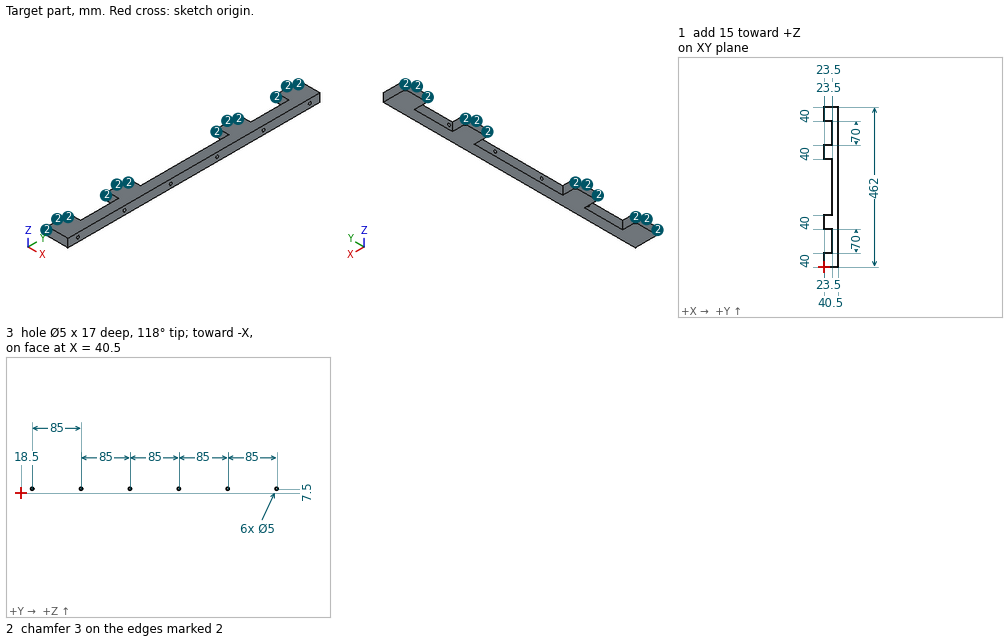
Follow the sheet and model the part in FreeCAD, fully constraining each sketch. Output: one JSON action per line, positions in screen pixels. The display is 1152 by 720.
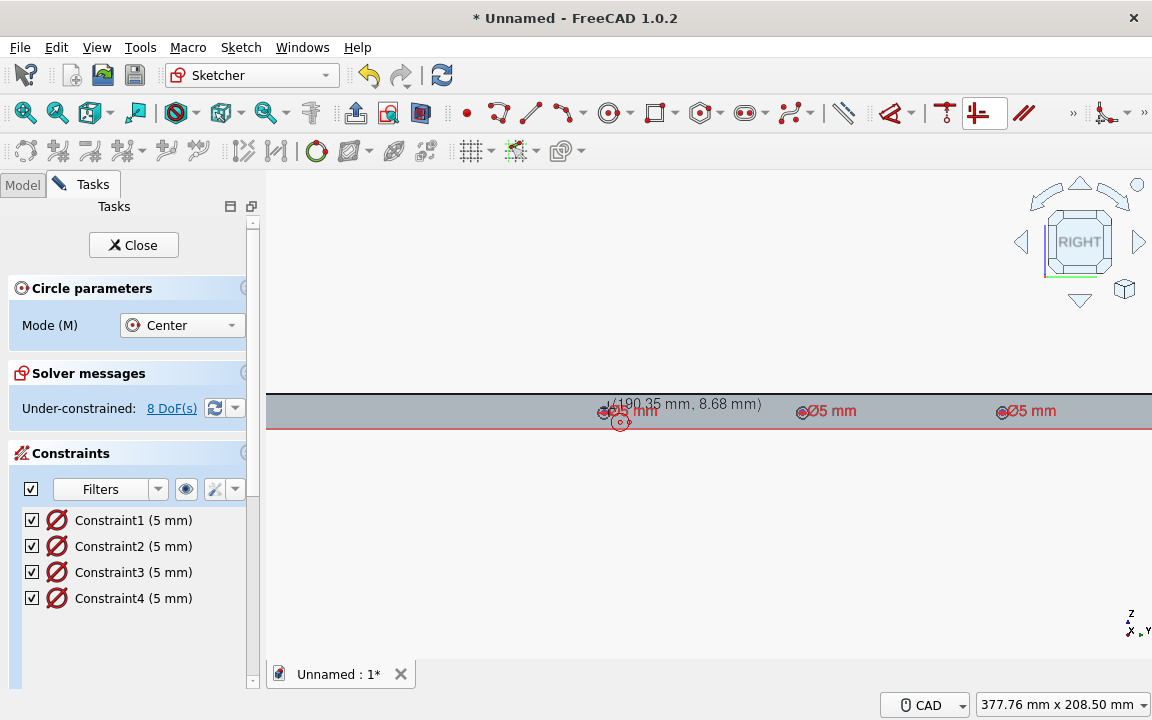
{"action": "scroll", "coordinate": [404, 412], "scroll_direction": "up", "scroll_amount": 7}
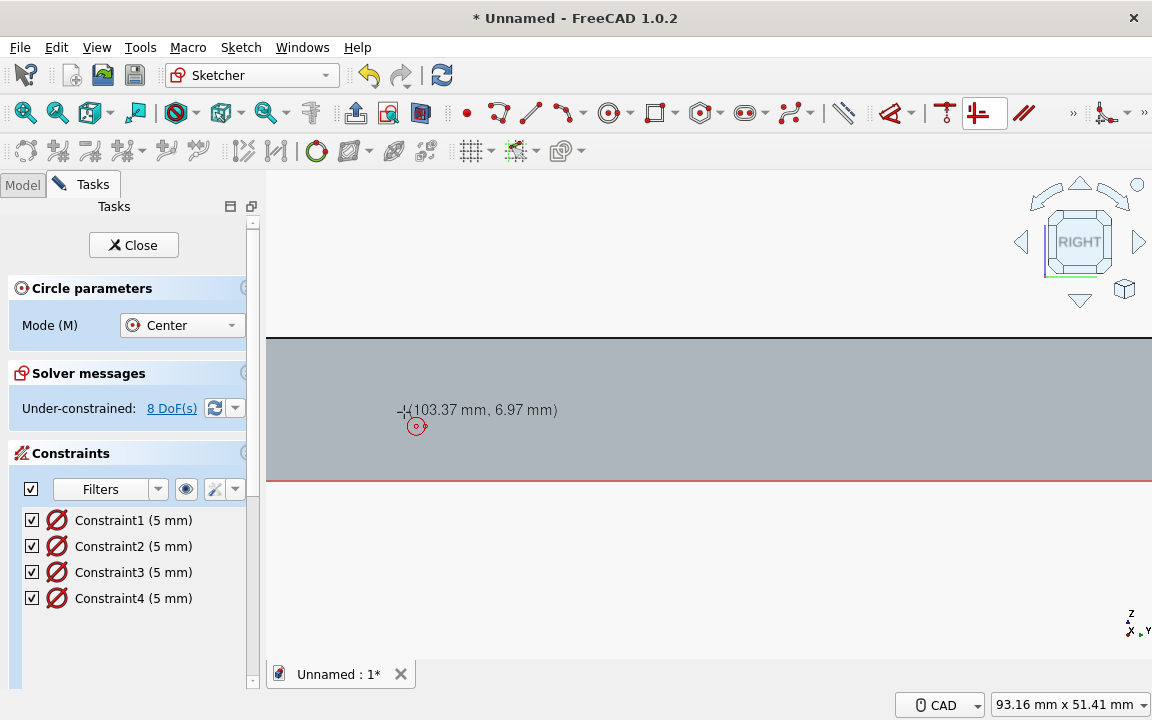
{"action": "scroll", "coordinate": [528, 412], "scroll_direction": "down", "scroll_amount": 11}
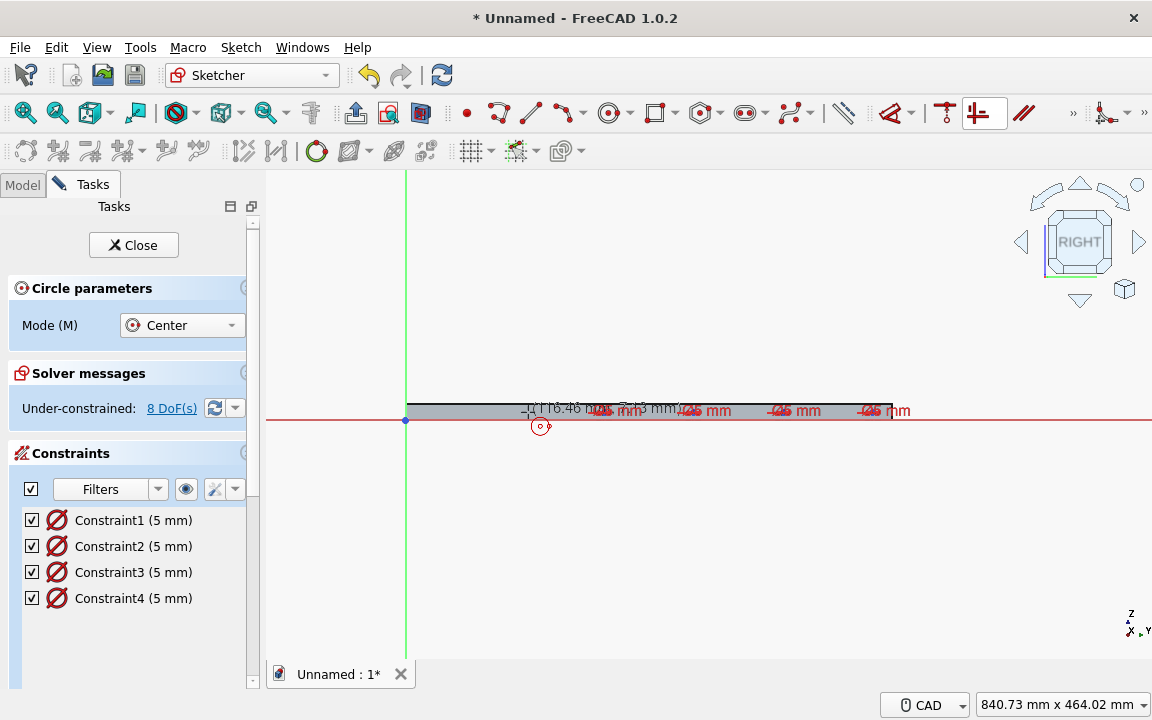
{"action": "scroll", "coordinate": [515, 412], "scroll_direction": "up", "scroll_amount": 4}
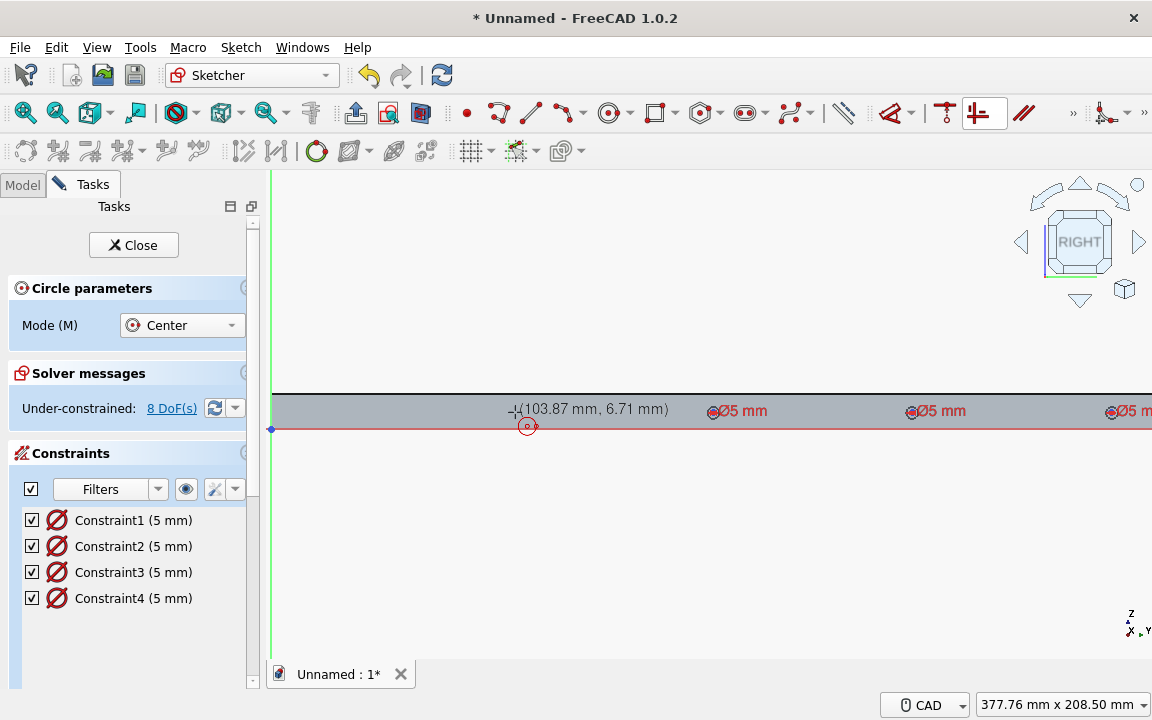
{"action": "left_click", "coordinate": [514, 412]}
{"action": "mouse_move", "coordinate": [518, 408]}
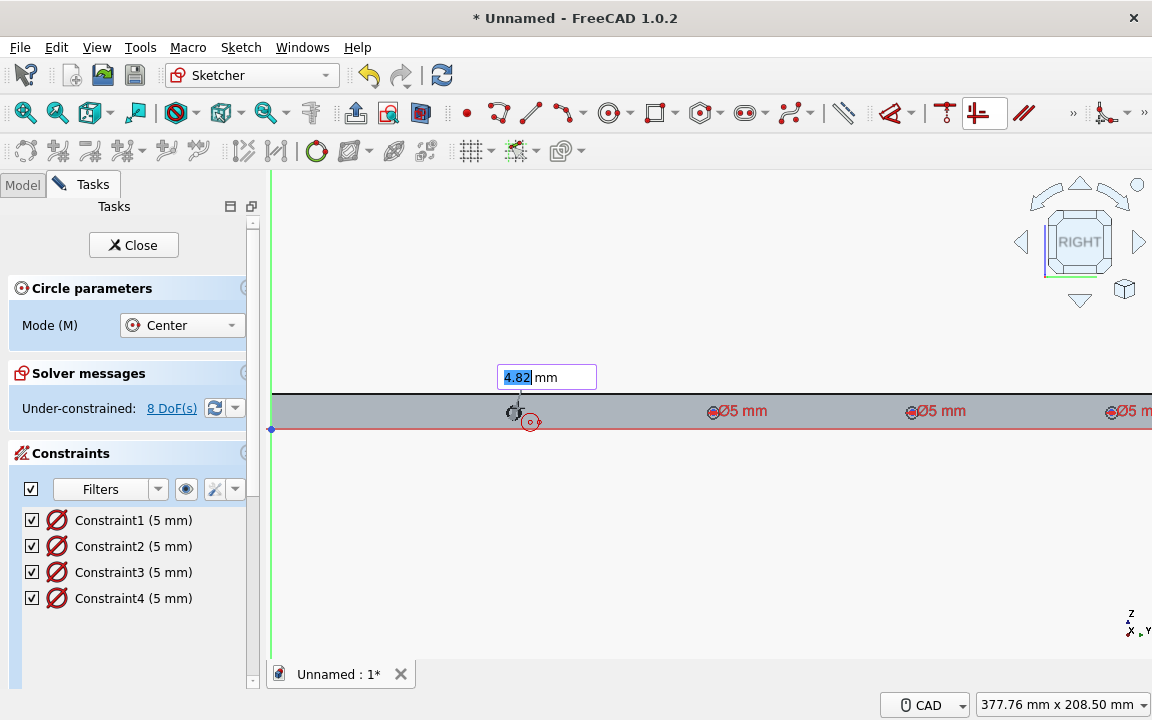
{"action": "type", "text": "5"}
{"action": "key", "text": "Return"}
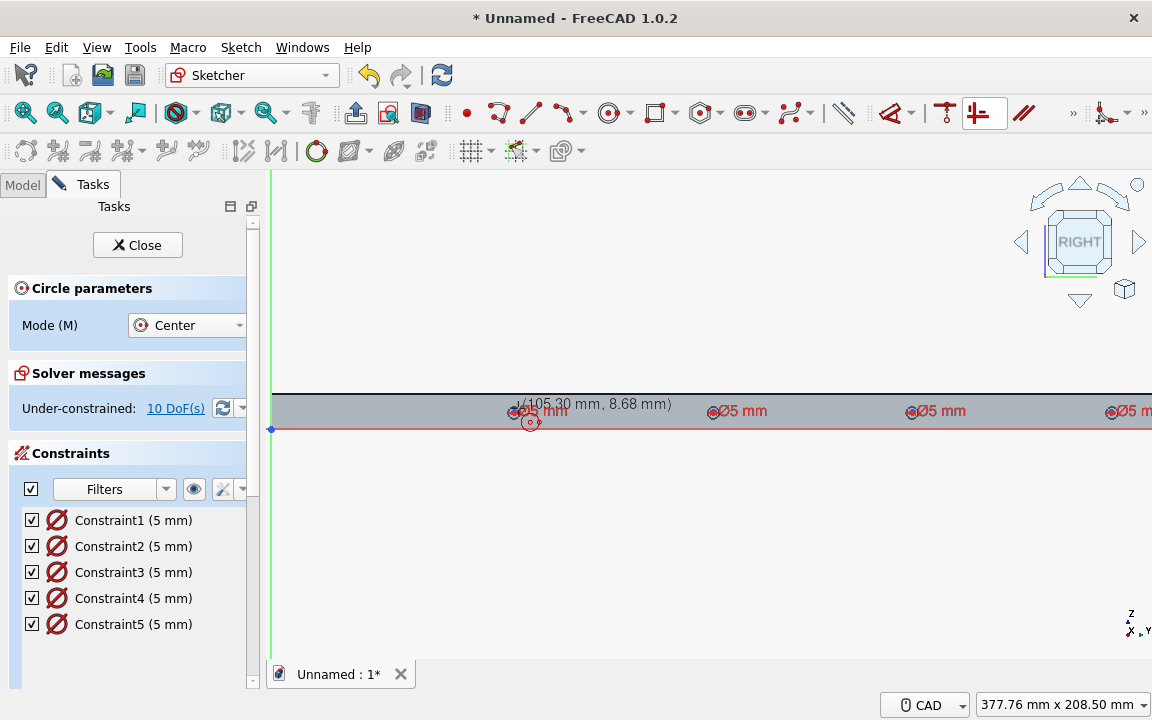
{"action": "scroll", "coordinate": [314, 412], "scroll_direction": "up", "scroll_amount": 7}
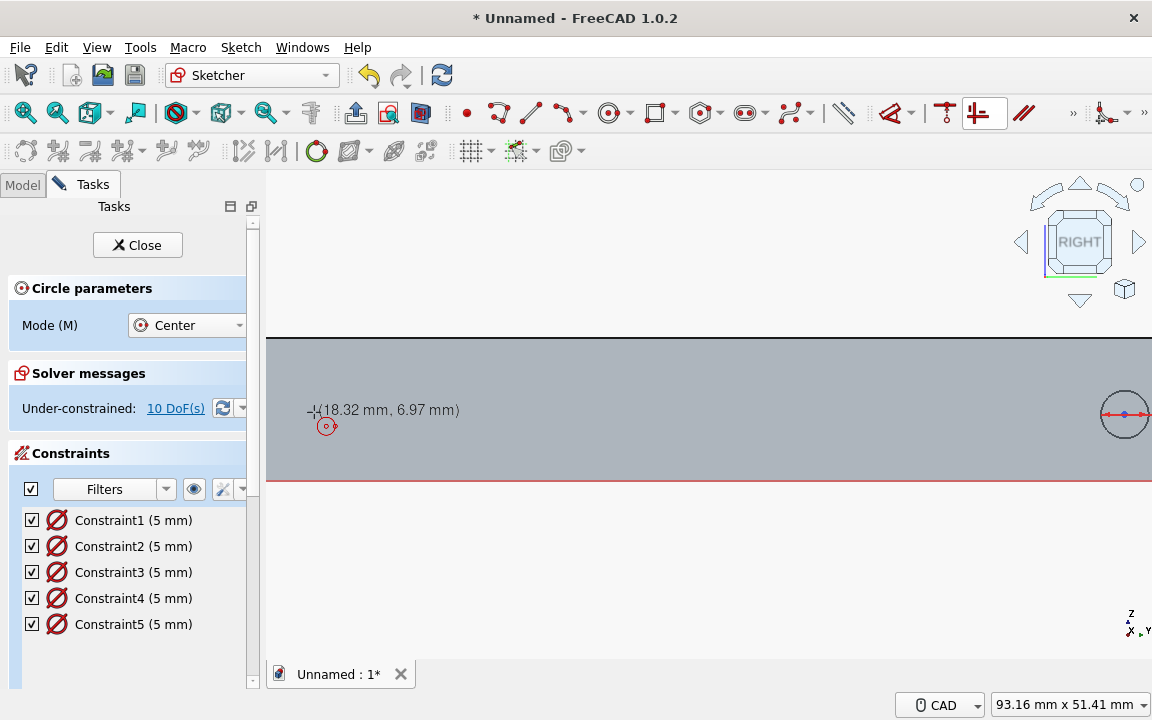
{"action": "scroll", "coordinate": [439, 412], "scroll_direction": "down", "scroll_amount": 11}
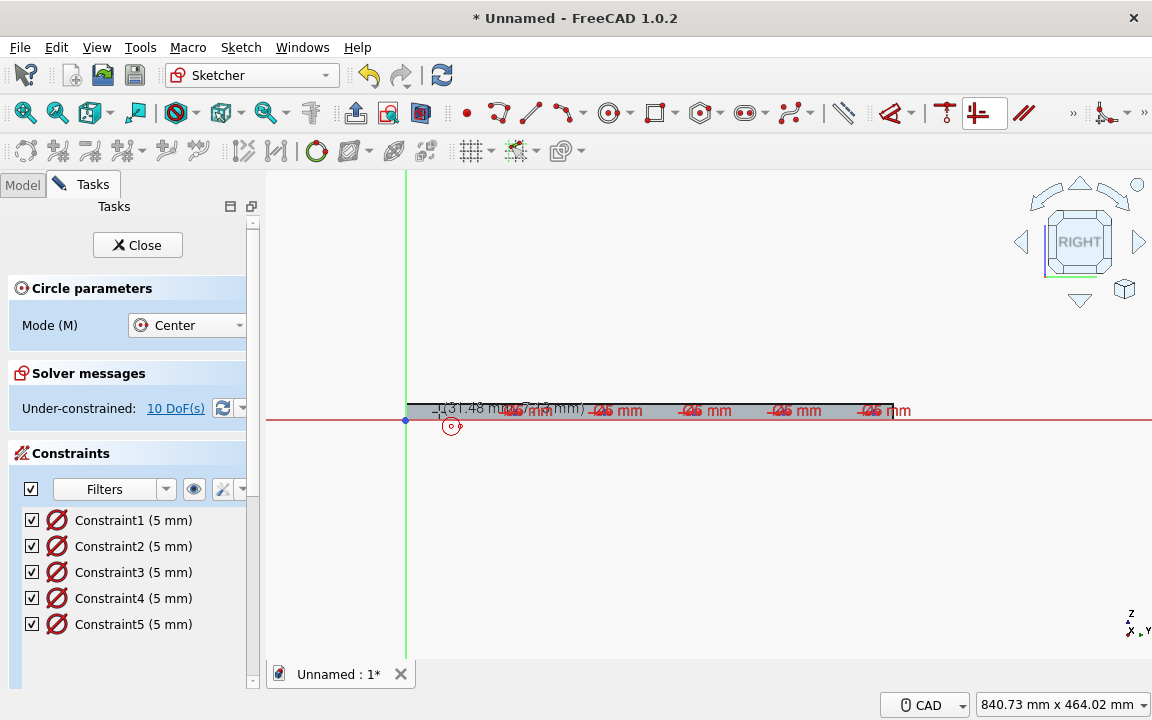
{"action": "scroll", "coordinate": [425, 412], "scroll_direction": "up", "scroll_amount": 4}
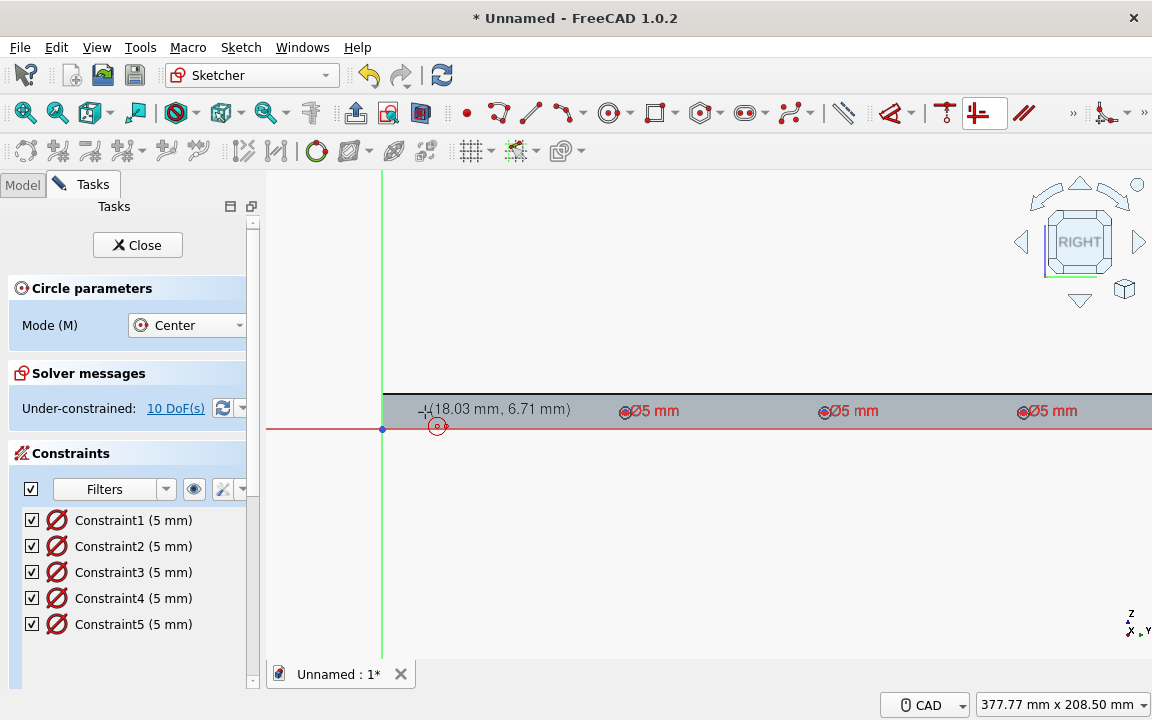
{"action": "left_click", "coordinate": [426, 412]}
{"action": "mouse_move", "coordinate": [430, 408]}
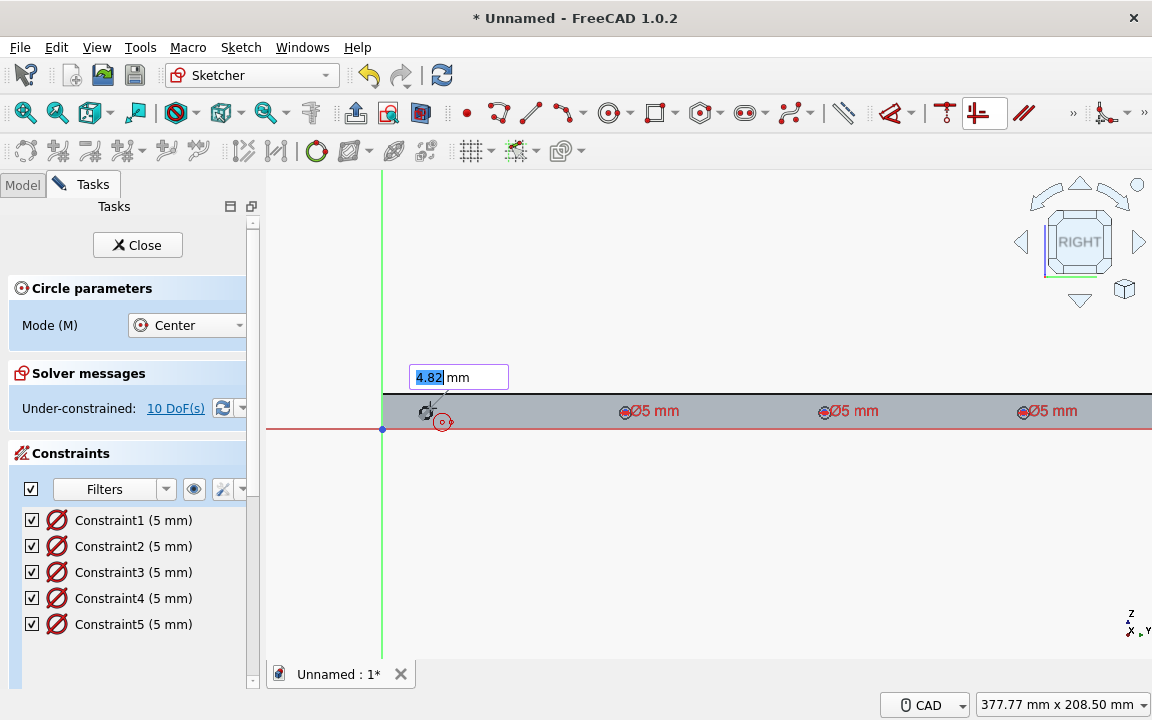
{"action": "type", "text": "5"}
{"action": "key", "text": "Return"}
{"action": "key", "text": "Escape"}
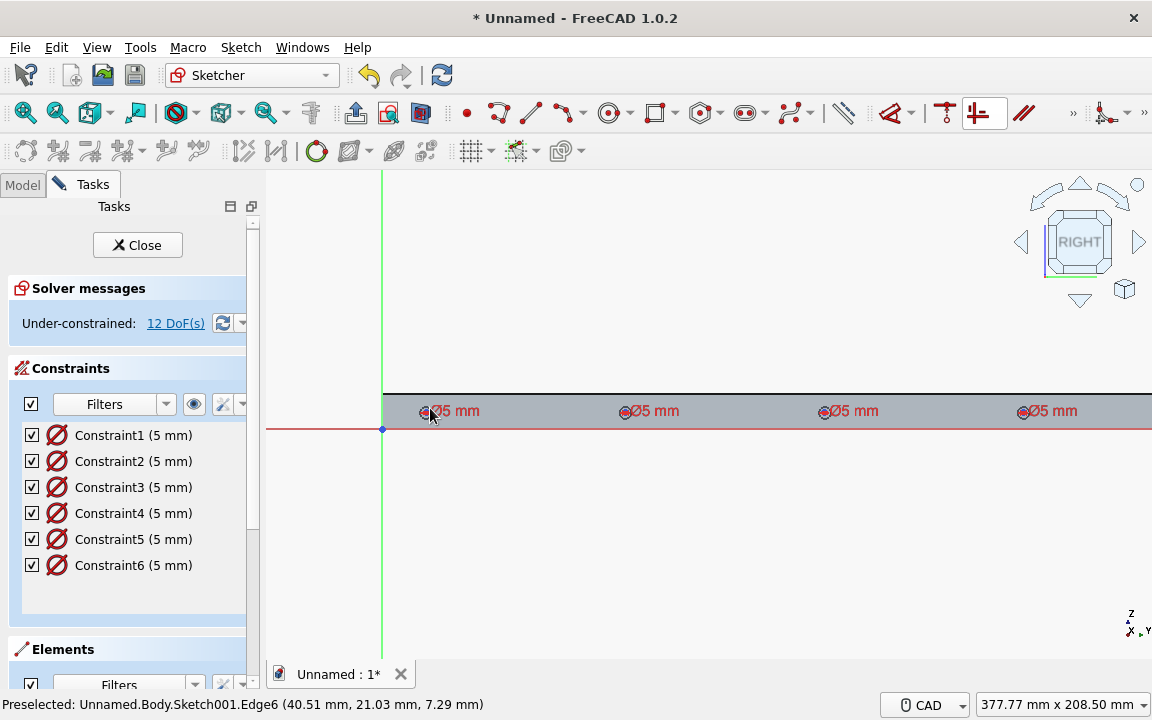
{"action": "scroll", "coordinate": [424, 412], "scroll_direction": "down", "scroll_amount": 4}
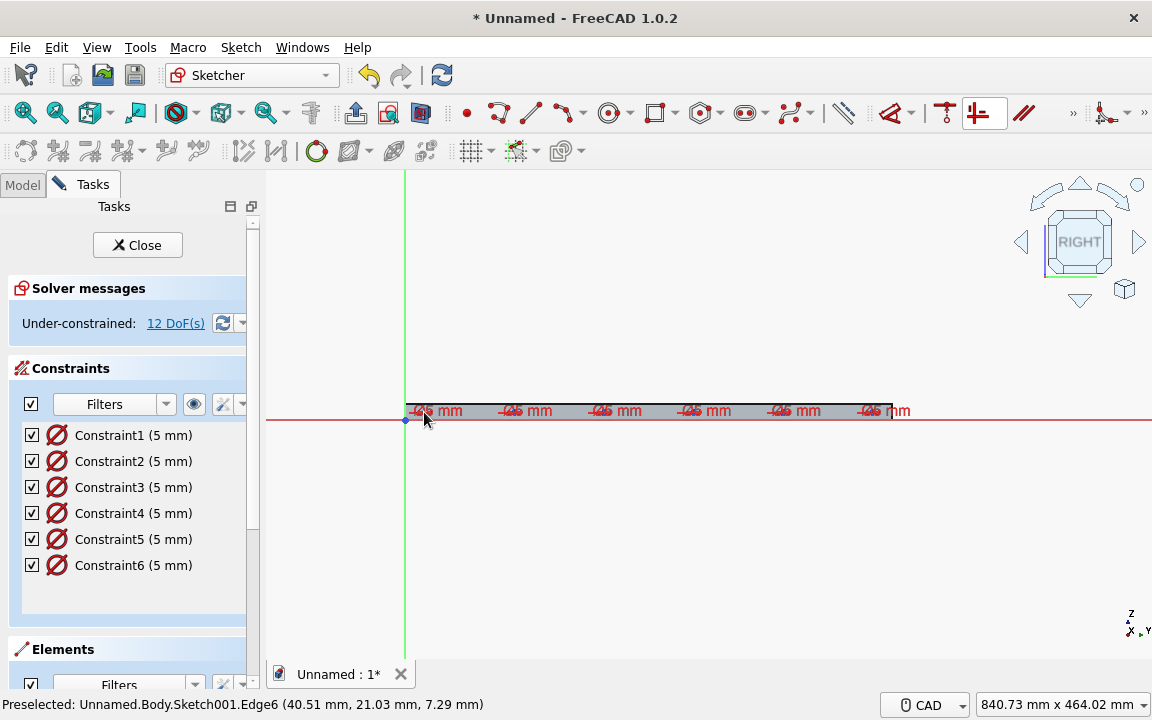
{"action": "left_click", "coordinate": [873, 413]}